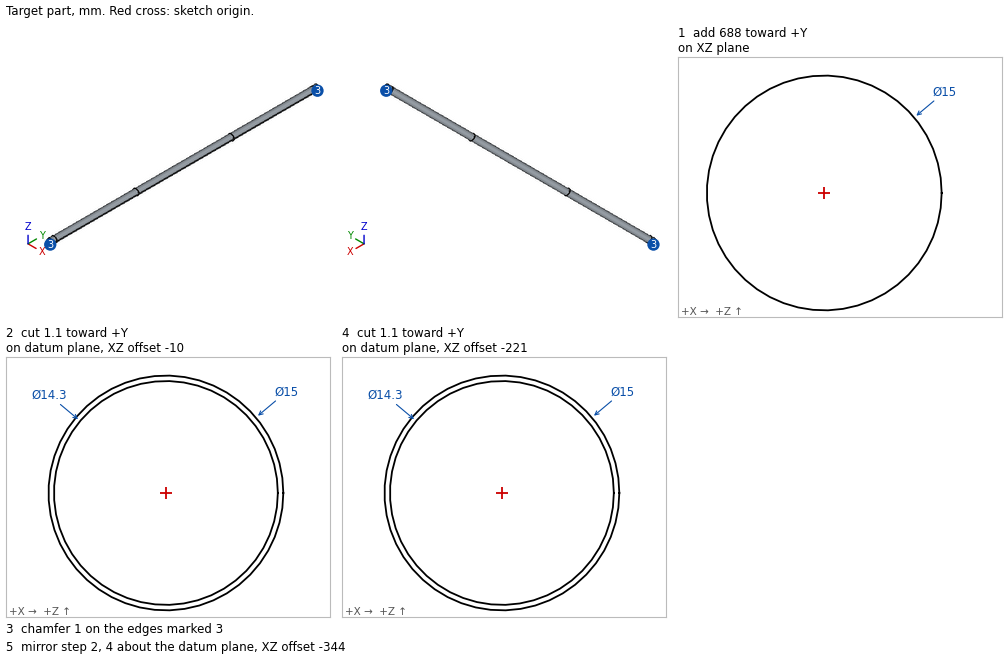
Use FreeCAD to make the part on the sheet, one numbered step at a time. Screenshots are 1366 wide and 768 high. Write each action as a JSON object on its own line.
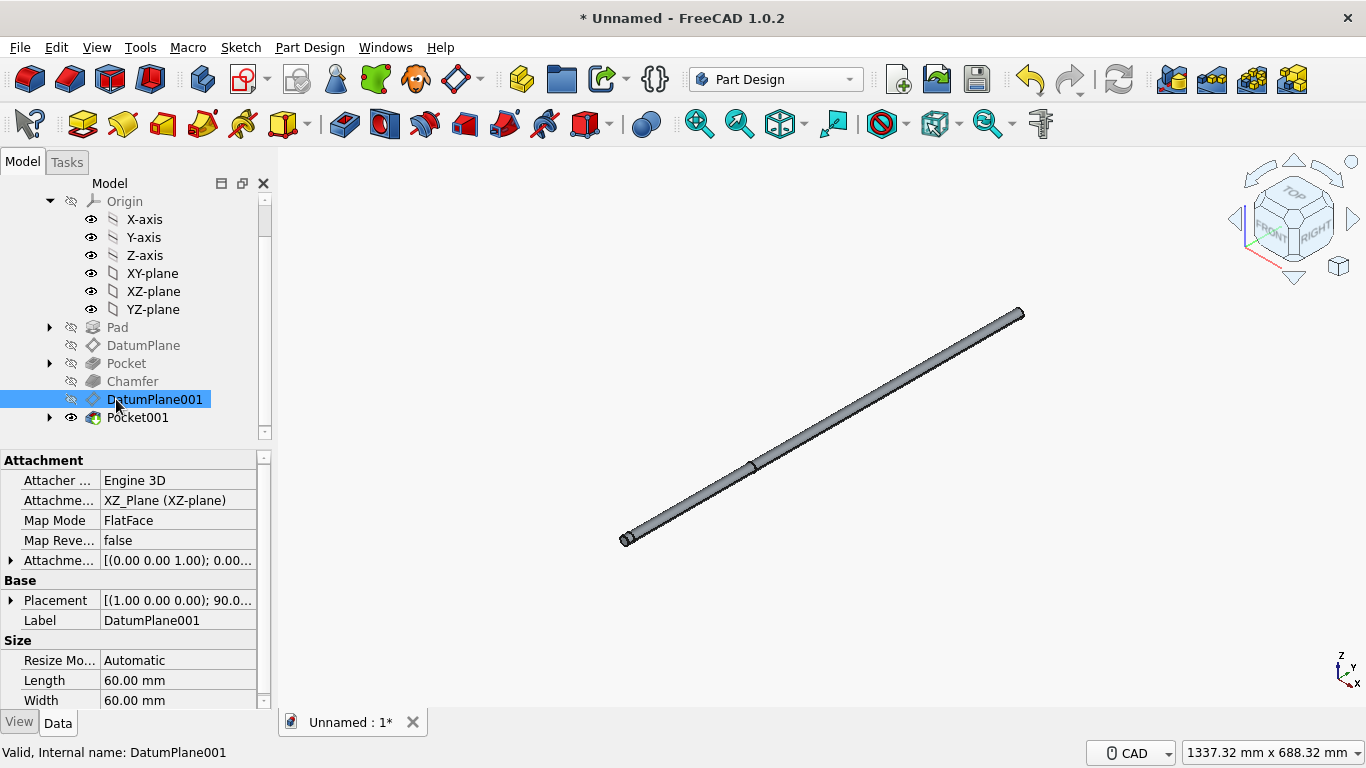
{"action": "left_click", "coordinate": [700, 124]}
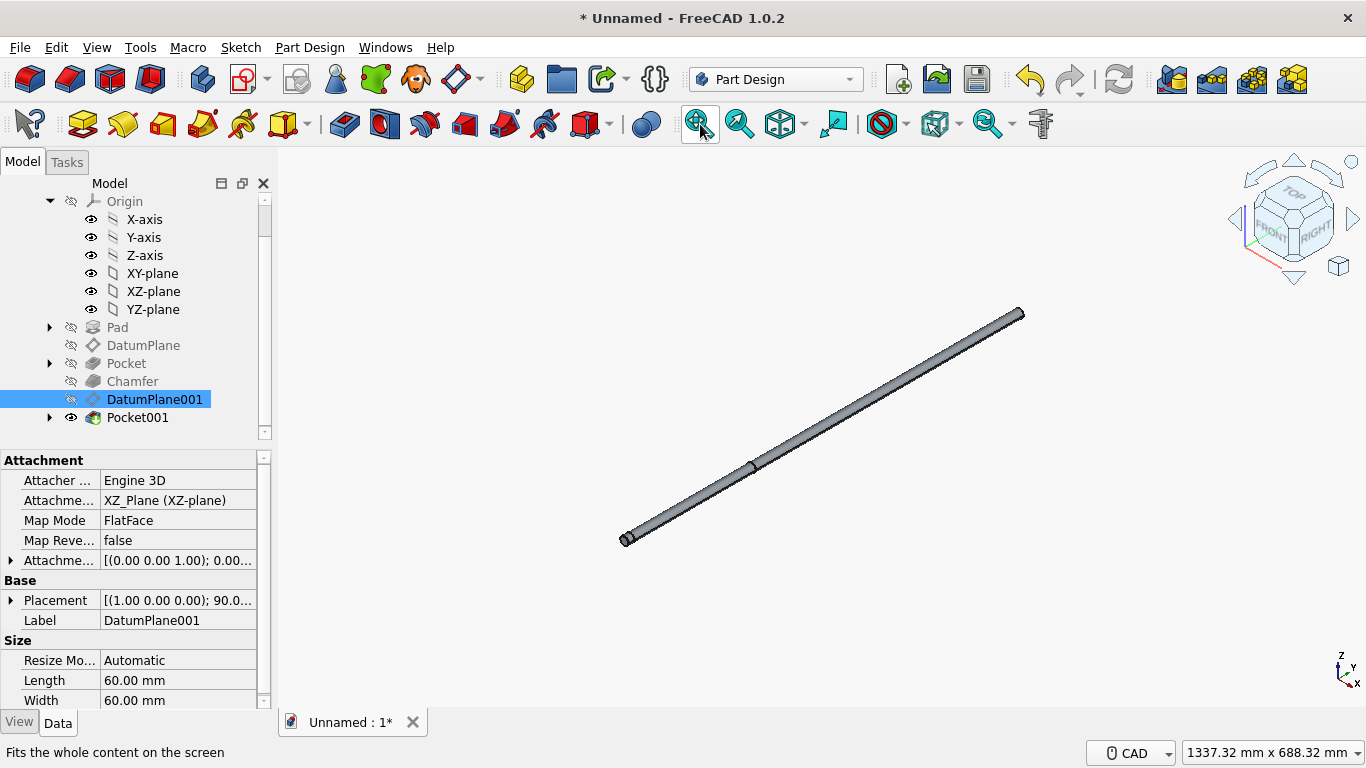
{"action": "left_click", "coordinate": [136, 291]}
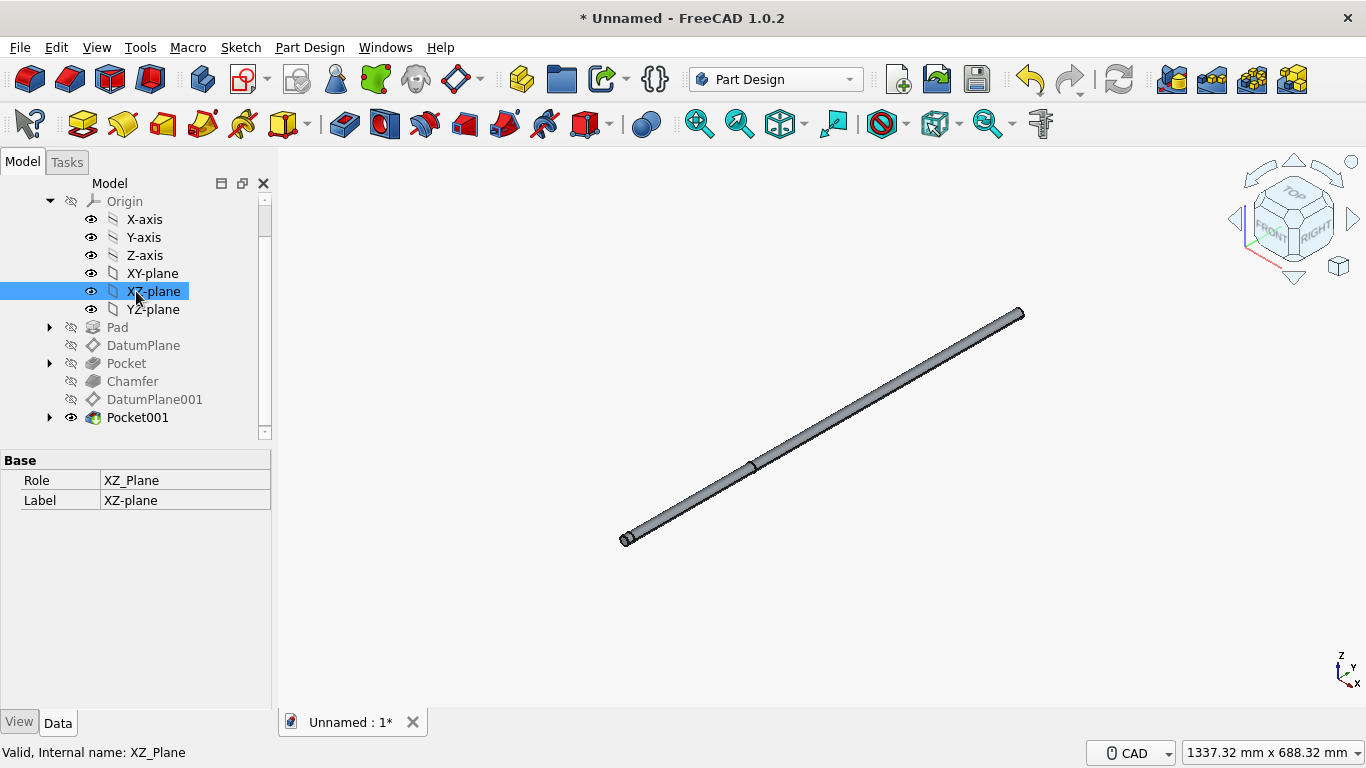
{"action": "left_click", "coordinate": [456, 80]}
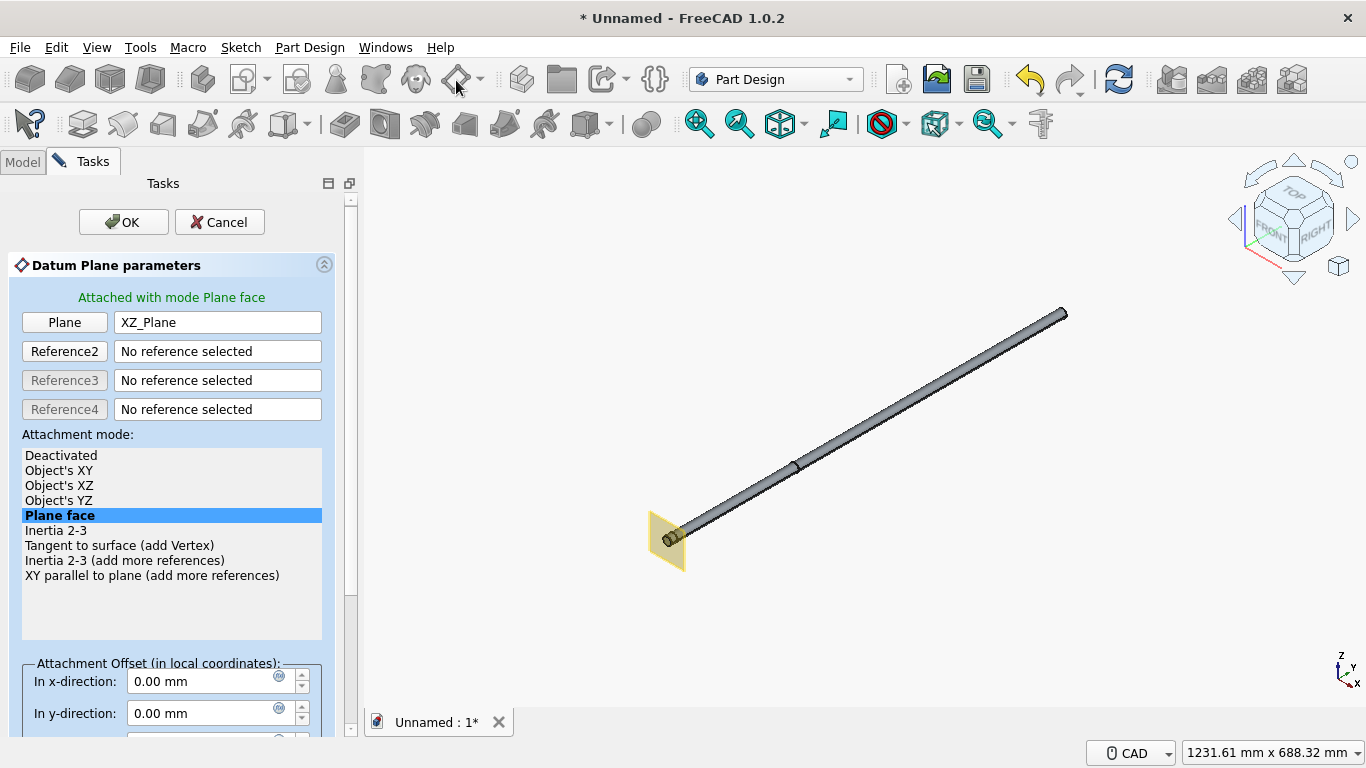
{"action": "scroll", "coordinate": [351, 464], "scroll_direction": "down", "scroll_amount": 2}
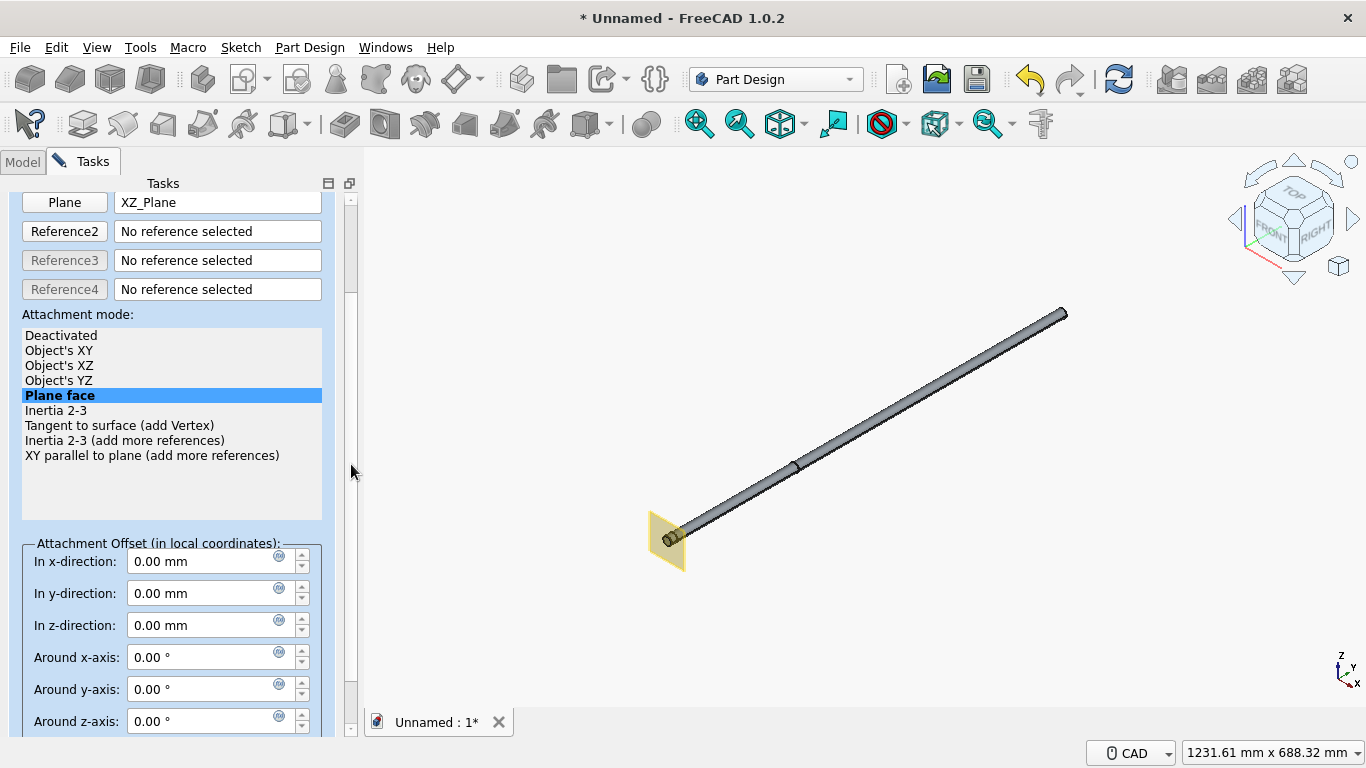
{"action": "triple_click", "coordinate": [210, 625]}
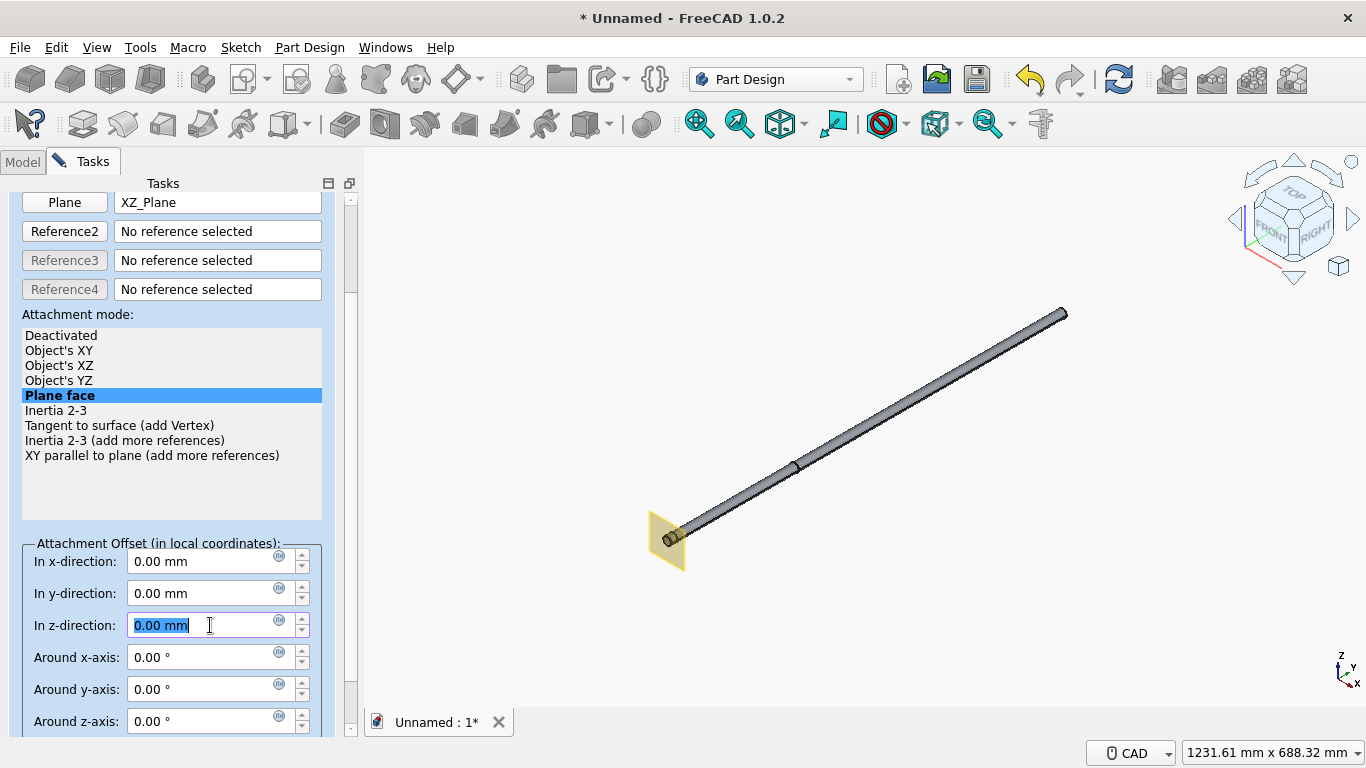
{"action": "type", "text": "-344"}
{"action": "key", "text": "Tab"}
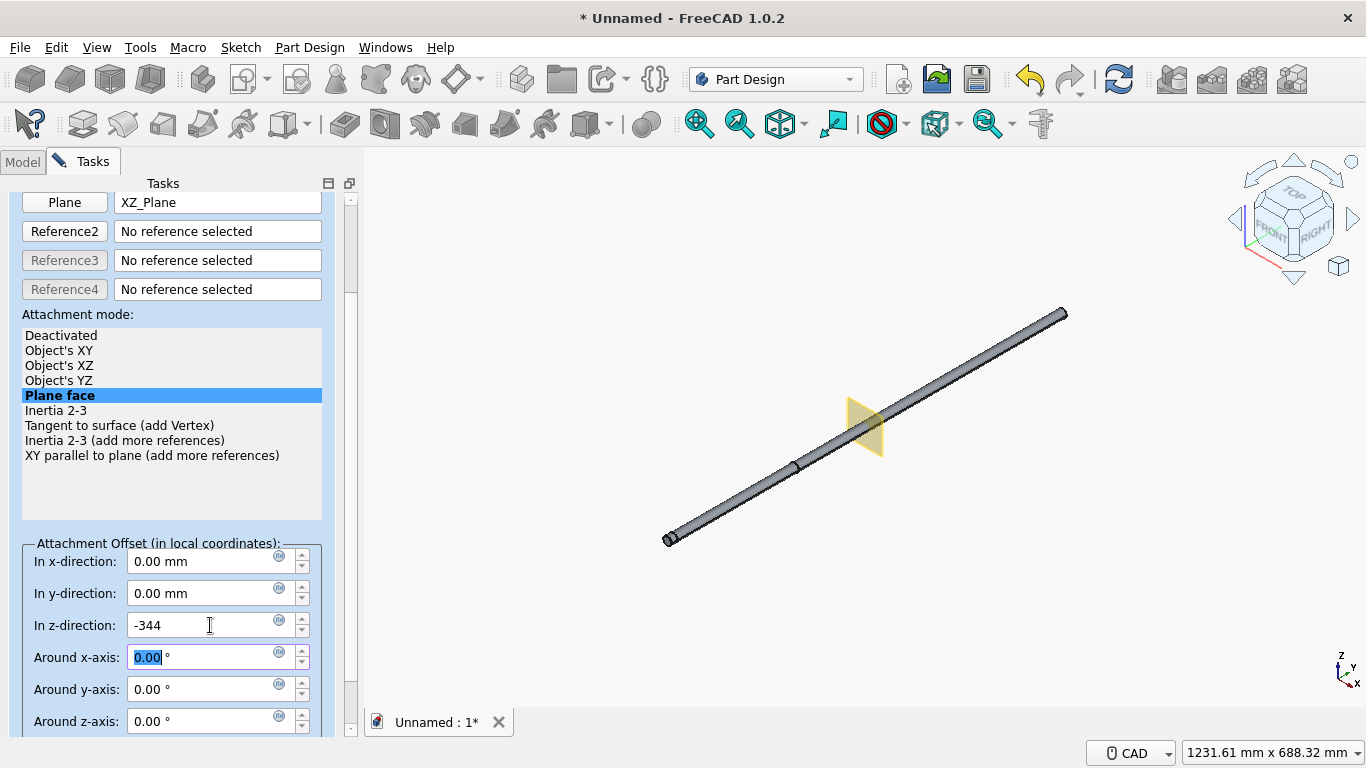
{"action": "scroll", "coordinate": [351, 464], "scroll_direction": "up", "scroll_amount": 3}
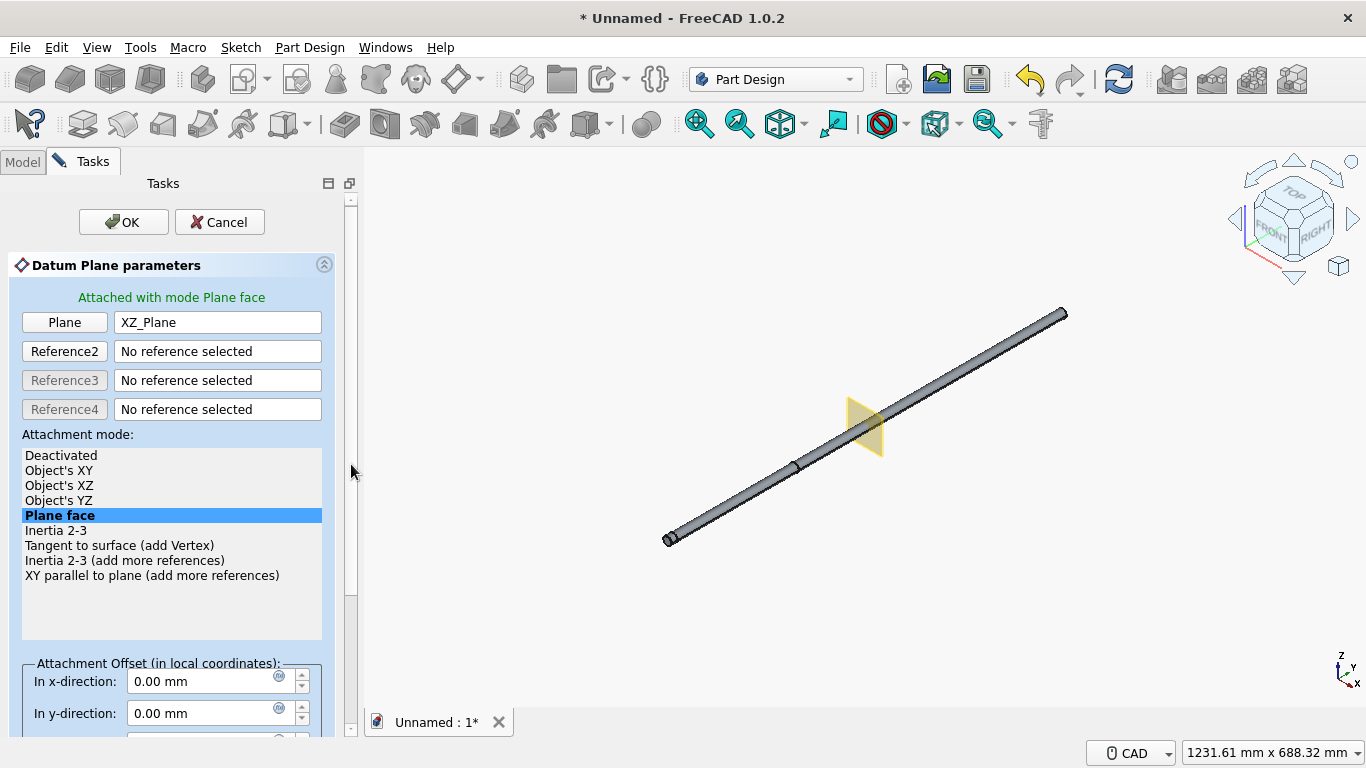
{"action": "left_click", "coordinate": [124, 222]}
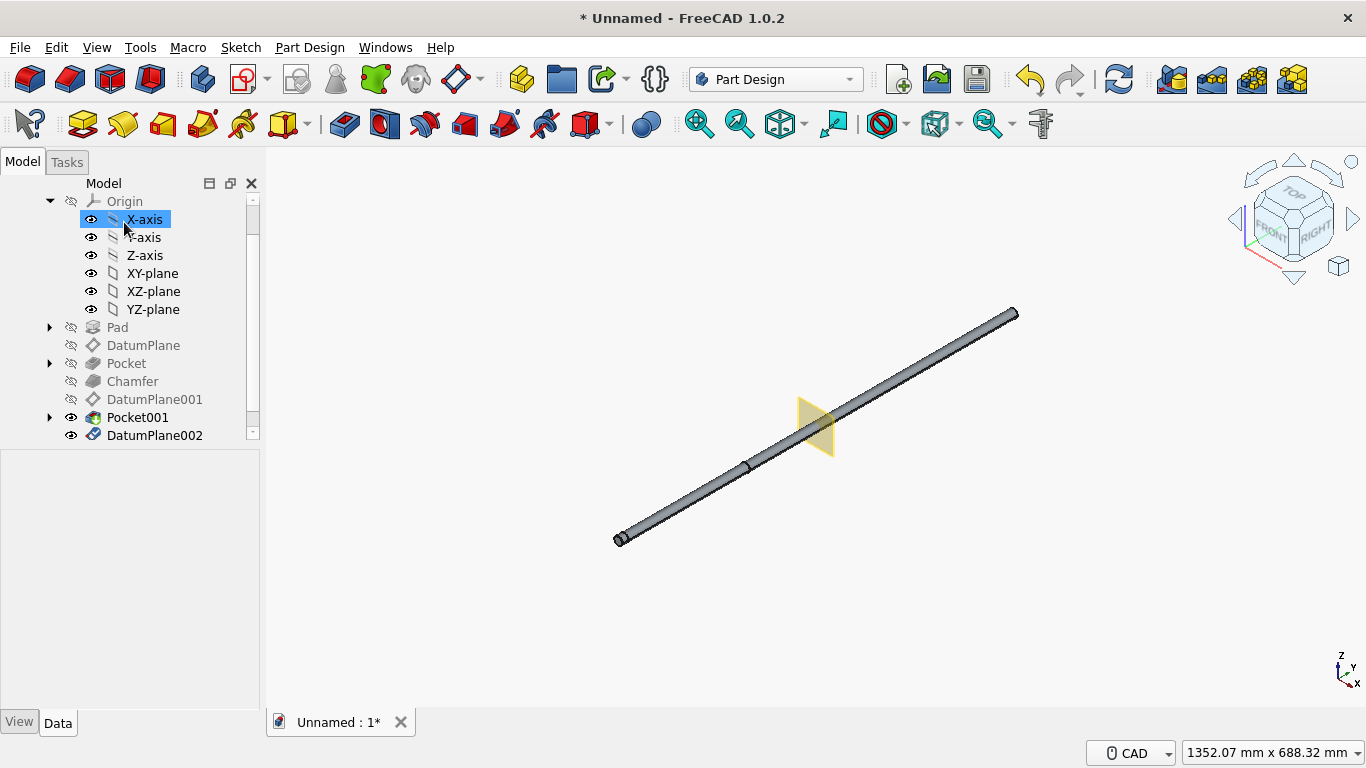
{"action": "left_click", "coordinate": [116, 363]}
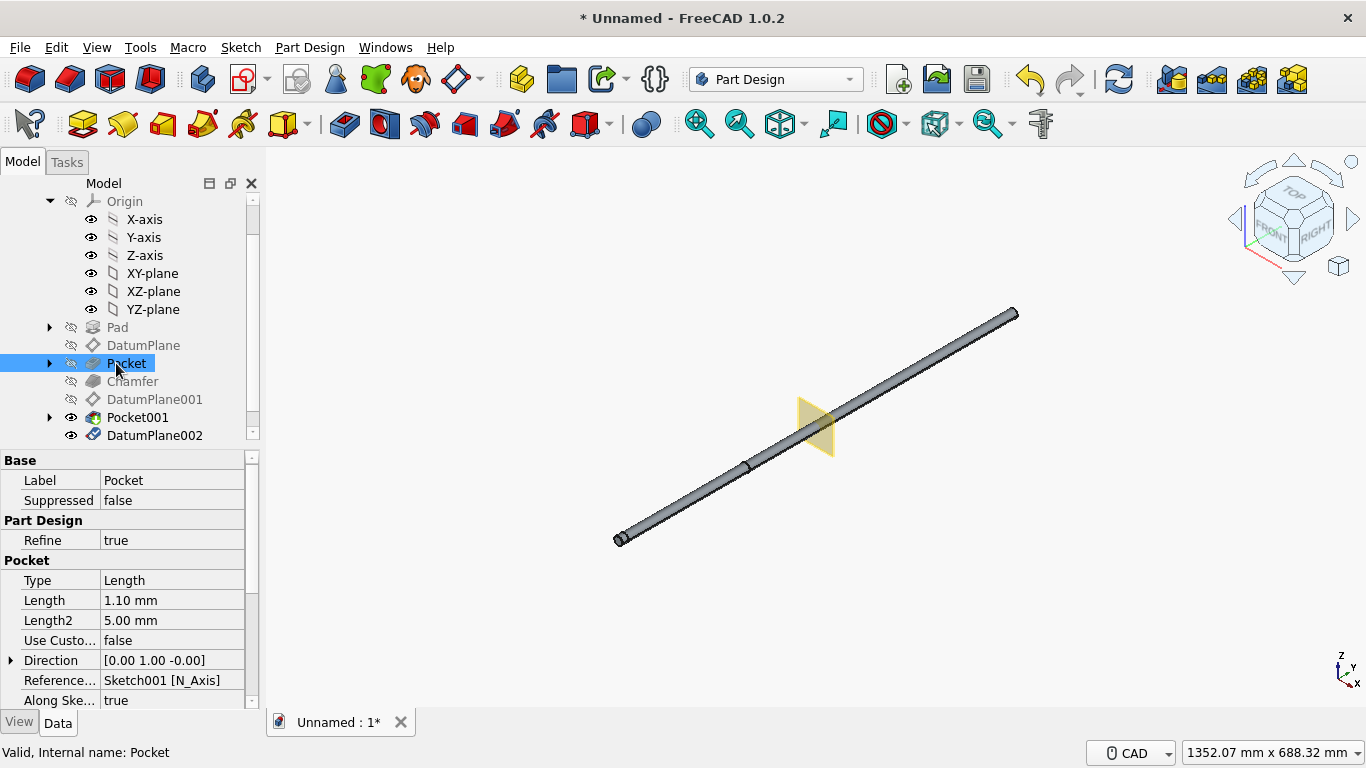
{"action": "left_click", "coordinate": [116, 417], "text": "ctrl"}